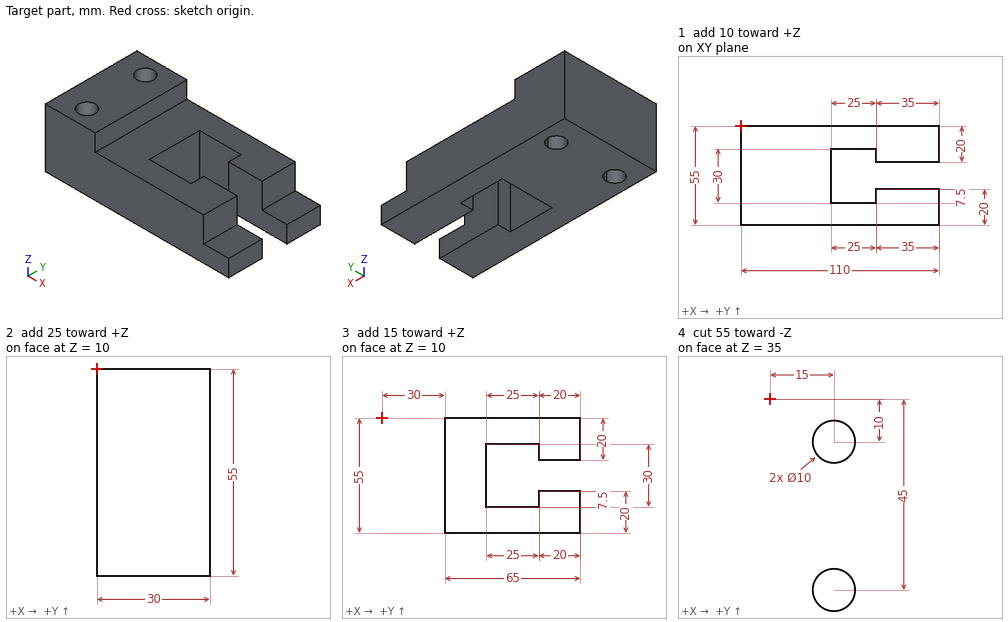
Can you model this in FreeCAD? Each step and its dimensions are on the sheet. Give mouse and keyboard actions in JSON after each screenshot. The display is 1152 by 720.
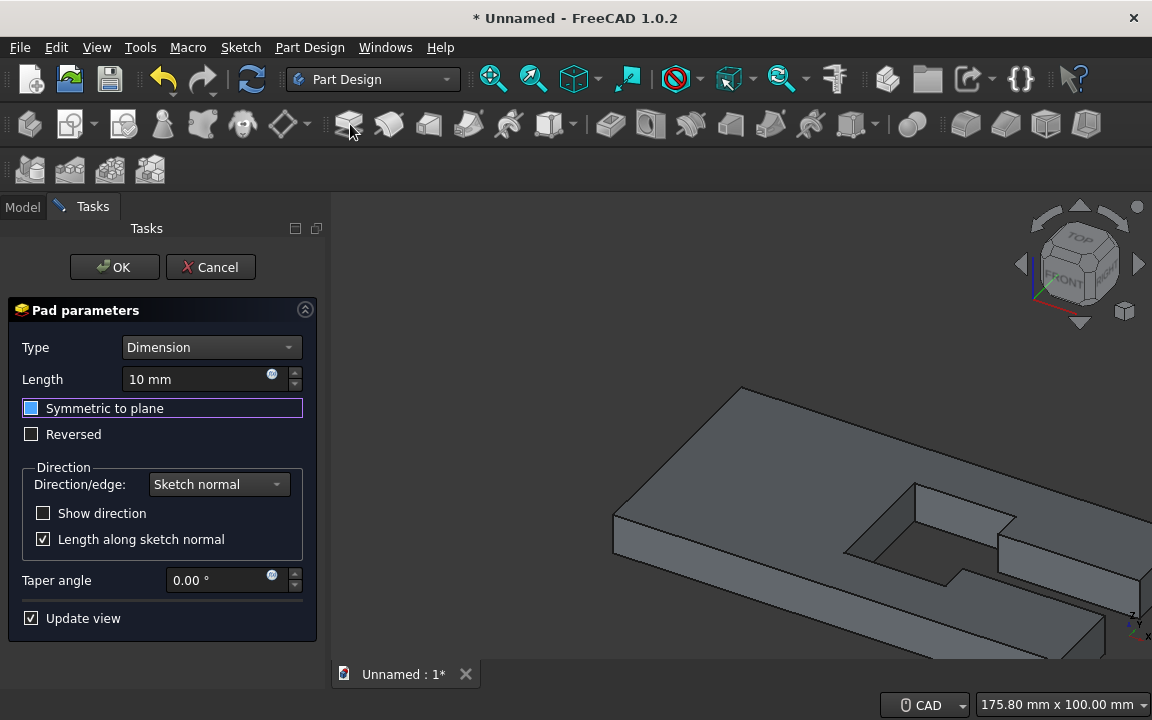
{"action": "left_click", "coordinate": [115, 267]}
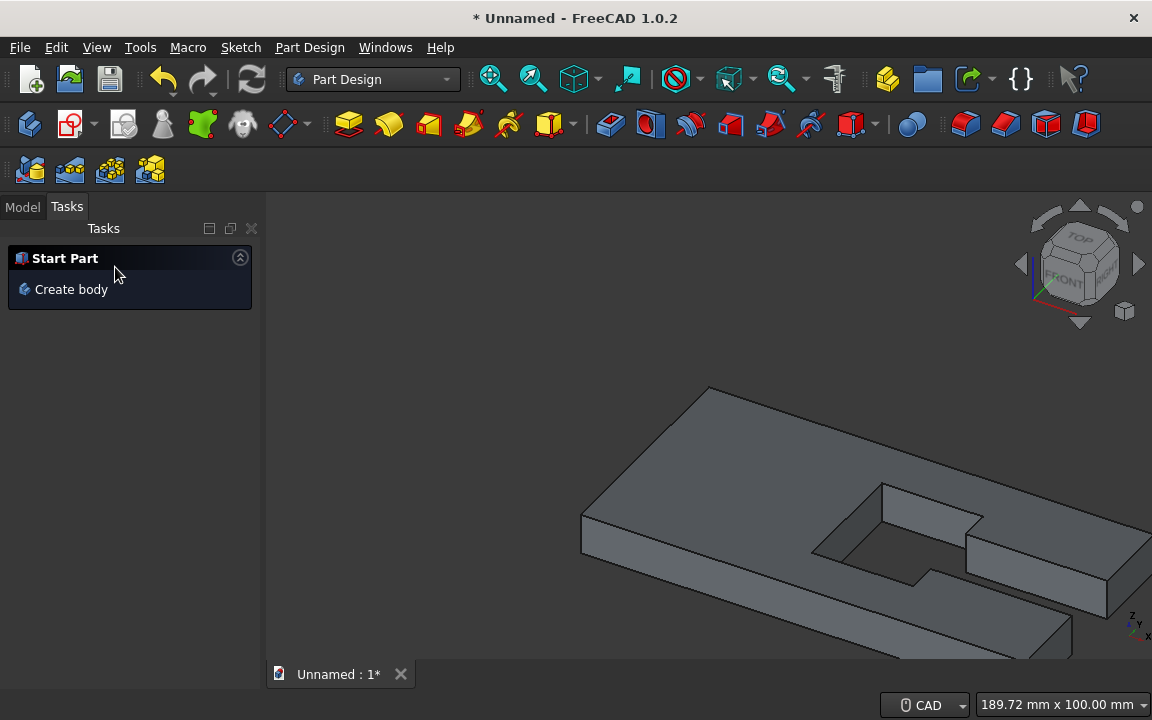
{"action": "left_click", "coordinate": [494, 80]}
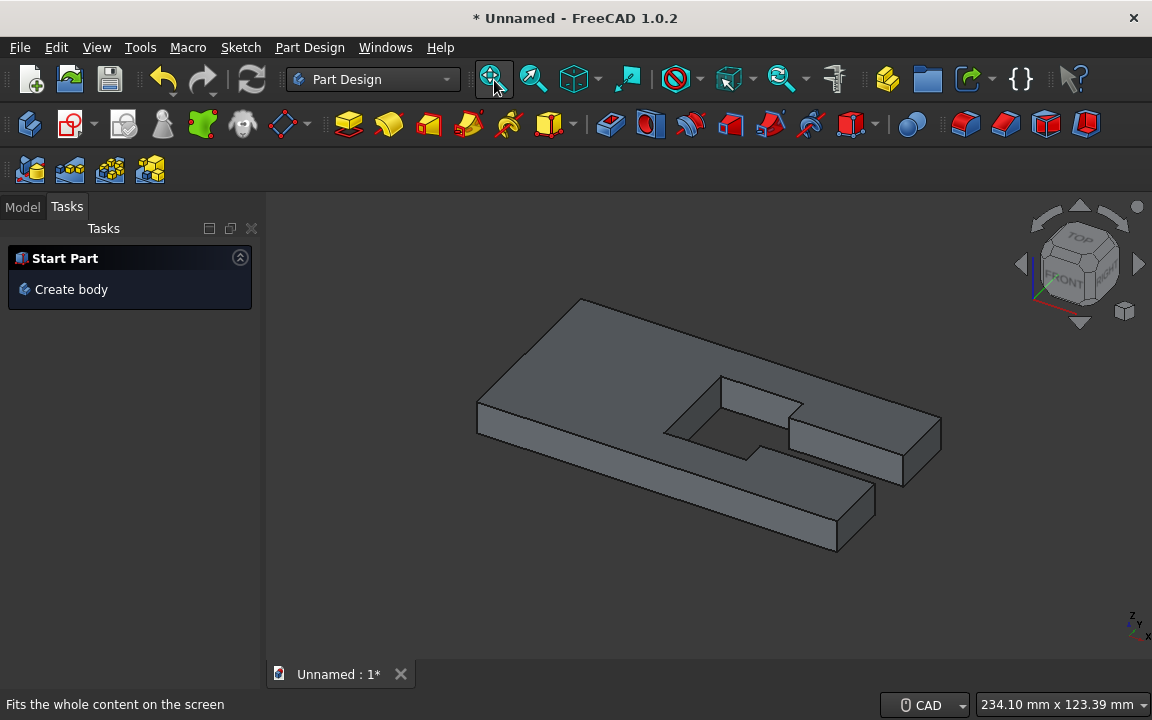
{"action": "left_click", "coordinate": [606, 375]}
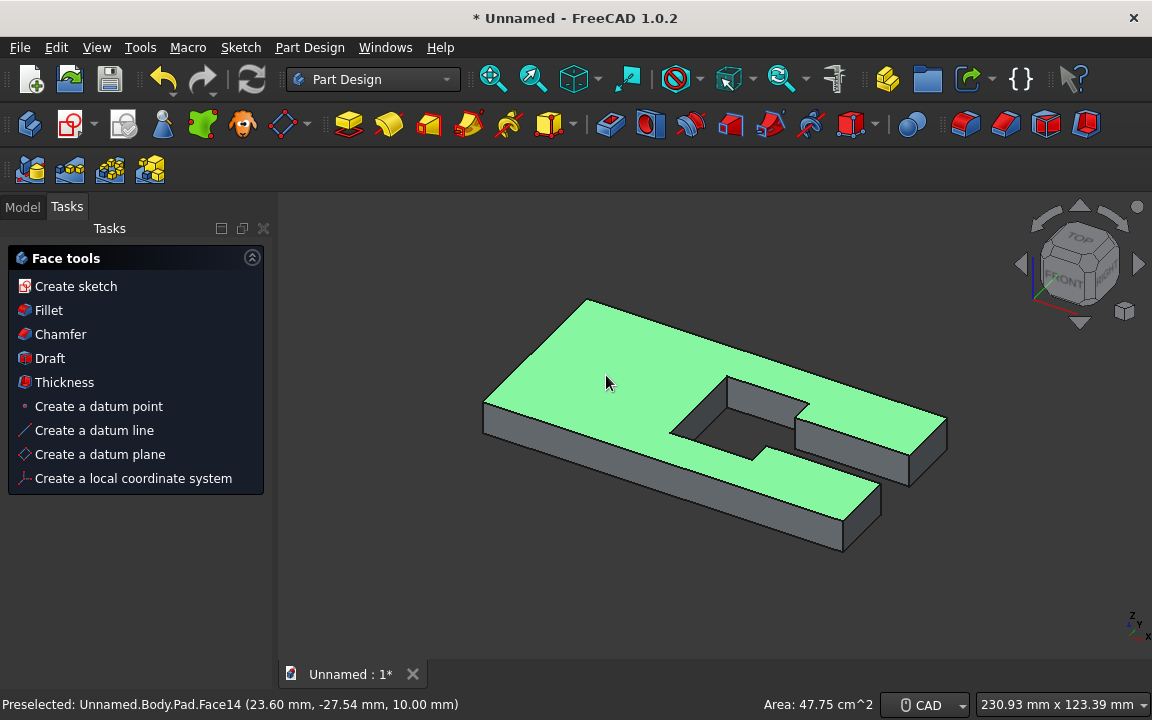
{"action": "left_click", "coordinate": [70, 124]}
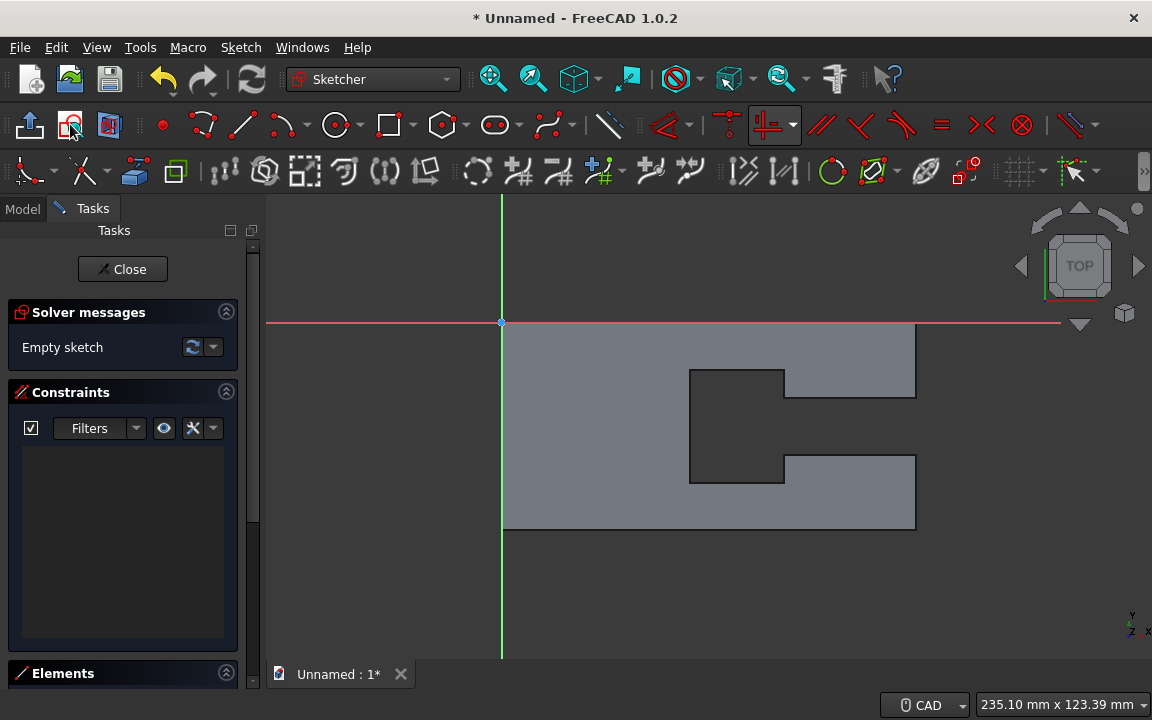
{"action": "scroll", "coordinate": [391, 426], "scroll_direction": "up", "scroll_amount": 2}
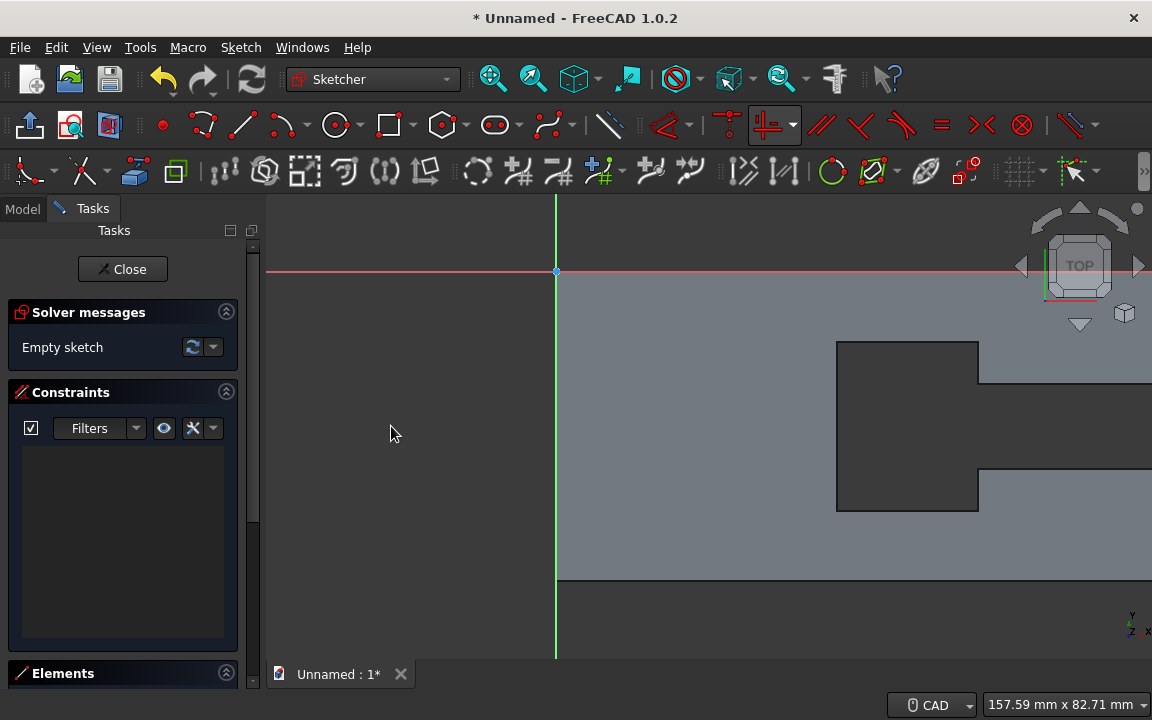
{"action": "left_click", "coordinate": [390, 126]}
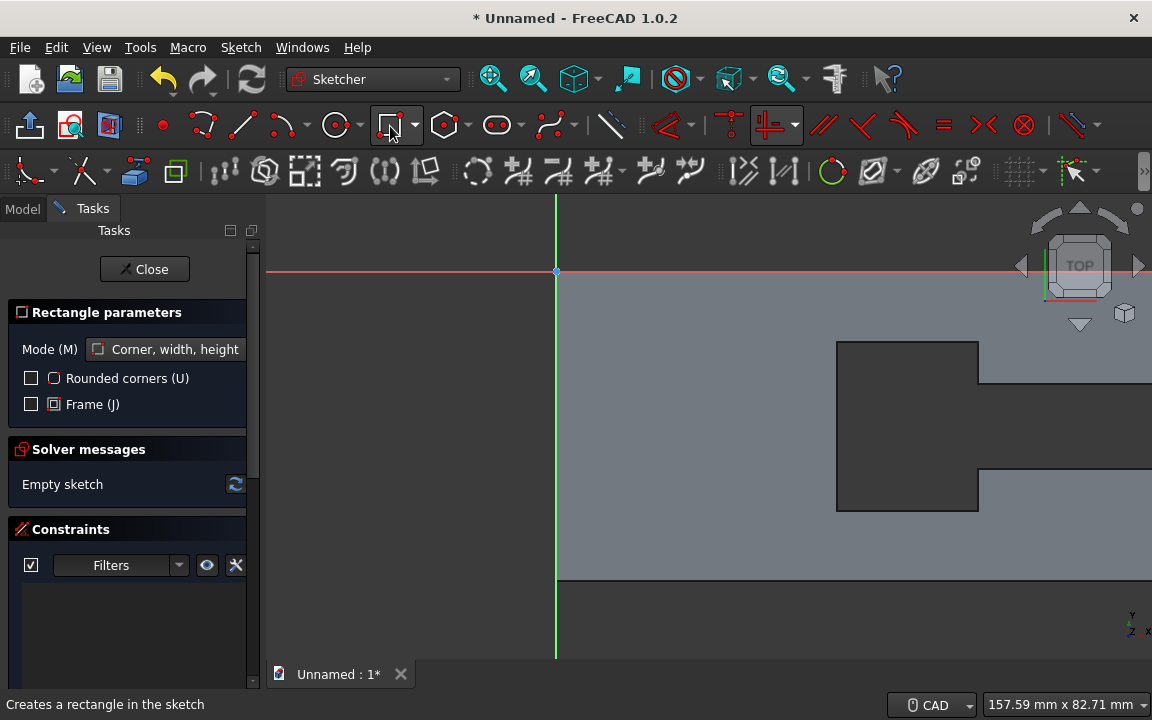
{"action": "left_click", "coordinate": [556, 272]}
{"action": "mouse_move", "coordinate": [725, 581]}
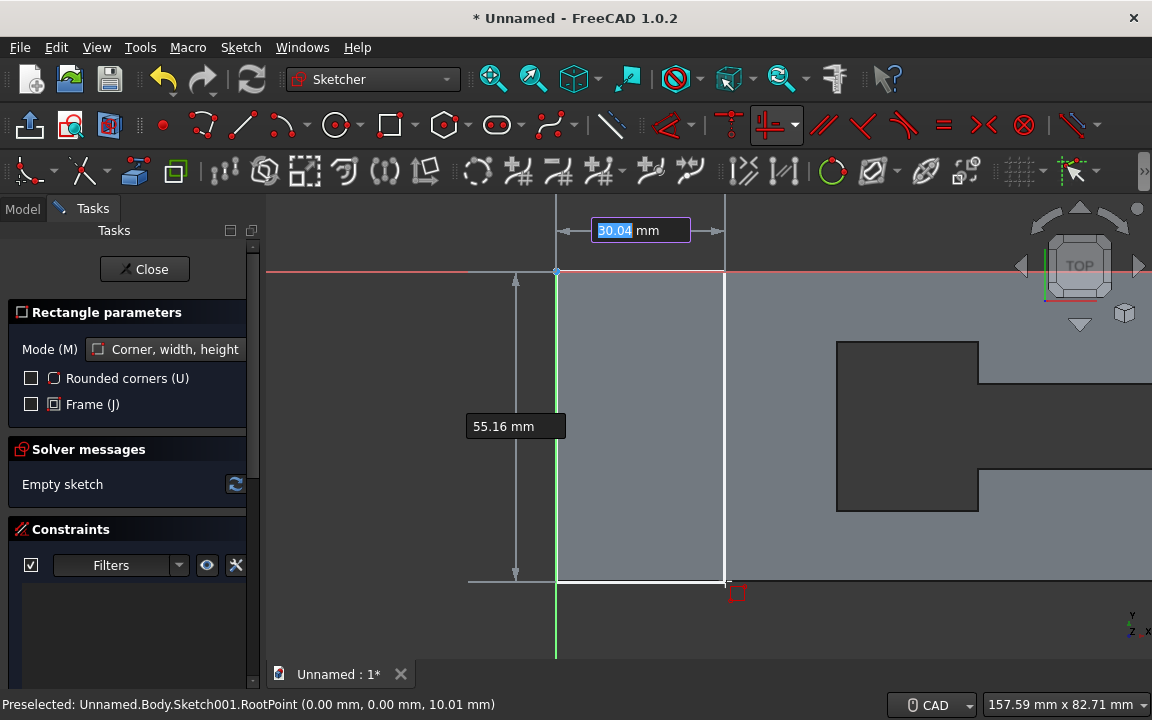
{"action": "type", "text": "30"}
{"action": "key", "text": "Tab"}
{"action": "type", "text": "55"}
{"action": "key", "text": "Return"}
{"action": "key", "text": "Escape"}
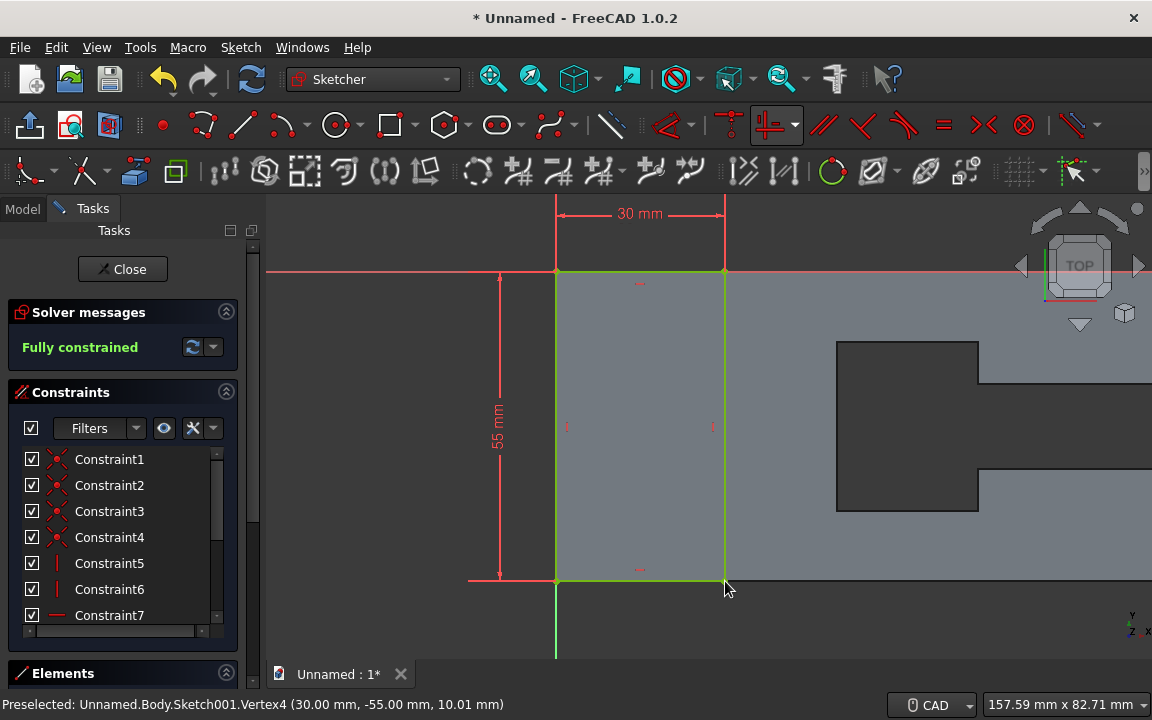
{"action": "left_click", "coordinate": [123, 269]}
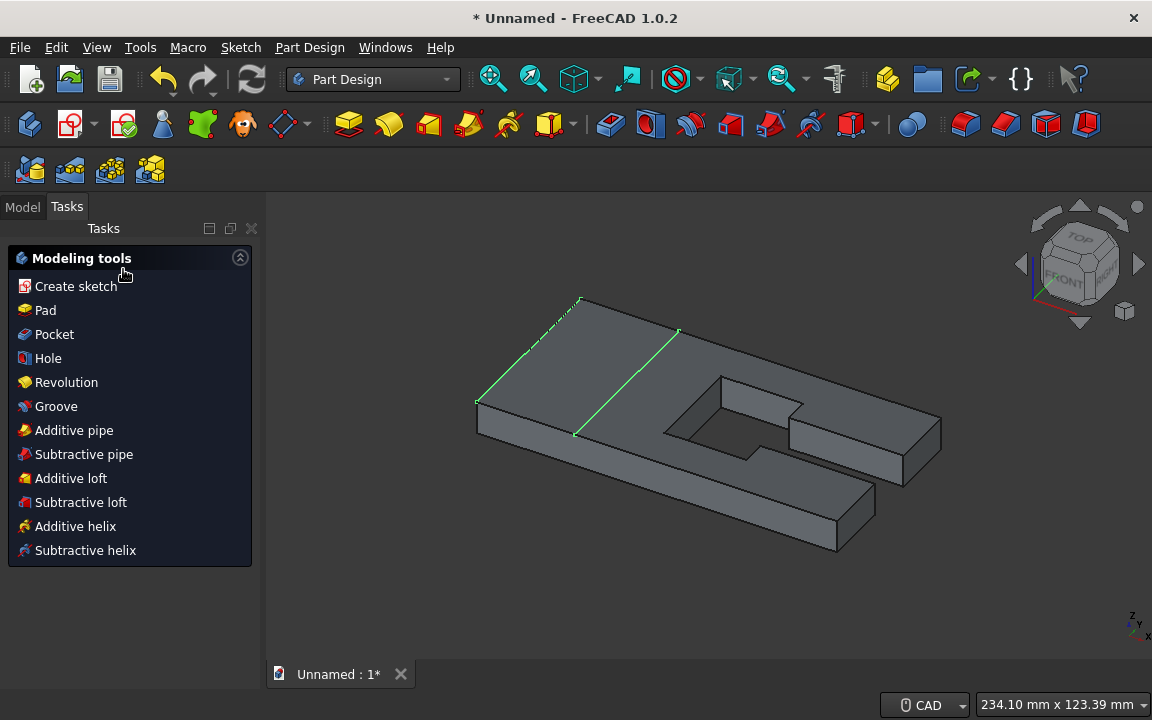
{"action": "left_click", "coordinate": [350, 124]}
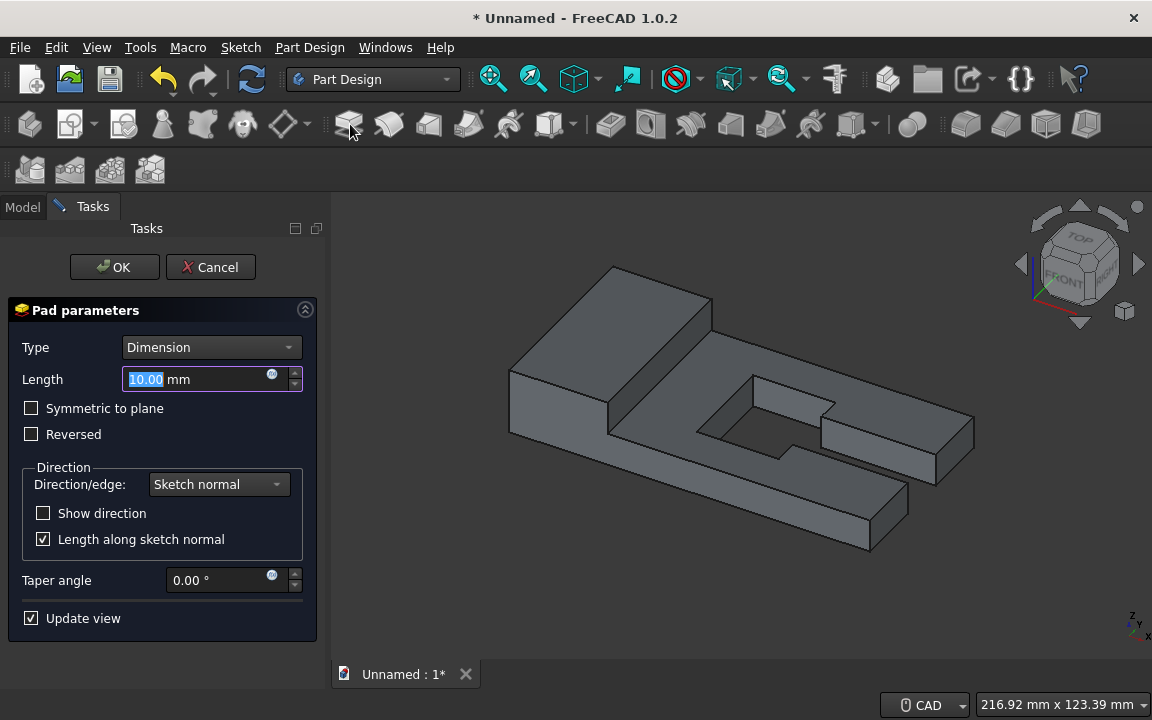
{"action": "type", "text": "25"}
{"action": "key", "text": "Tab"}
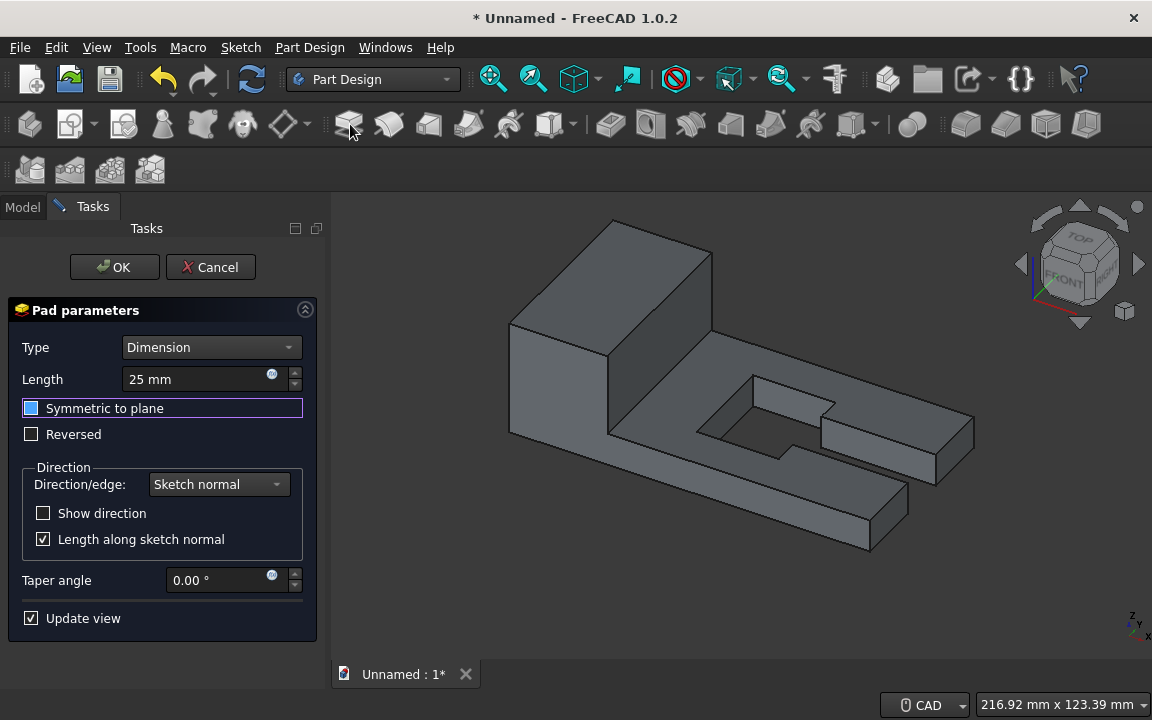
{"action": "left_click", "coordinate": [115, 267]}